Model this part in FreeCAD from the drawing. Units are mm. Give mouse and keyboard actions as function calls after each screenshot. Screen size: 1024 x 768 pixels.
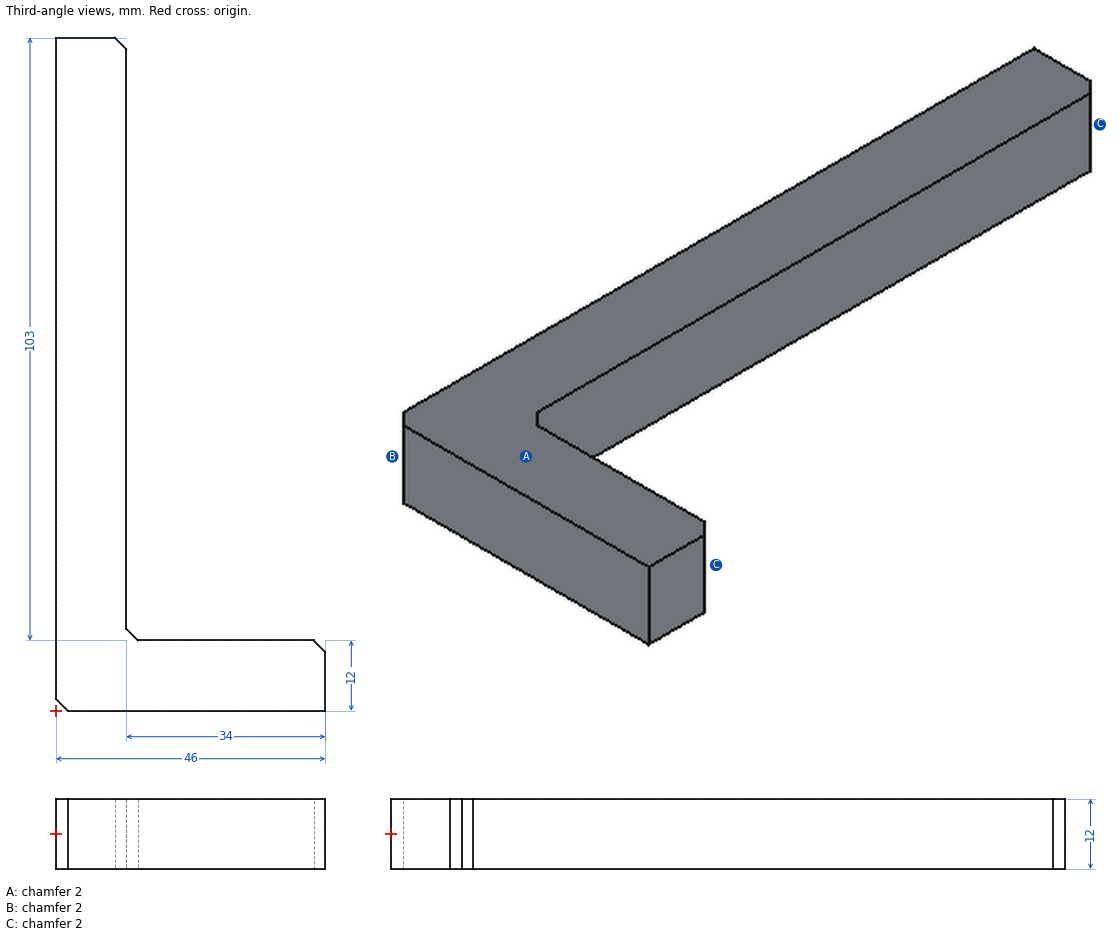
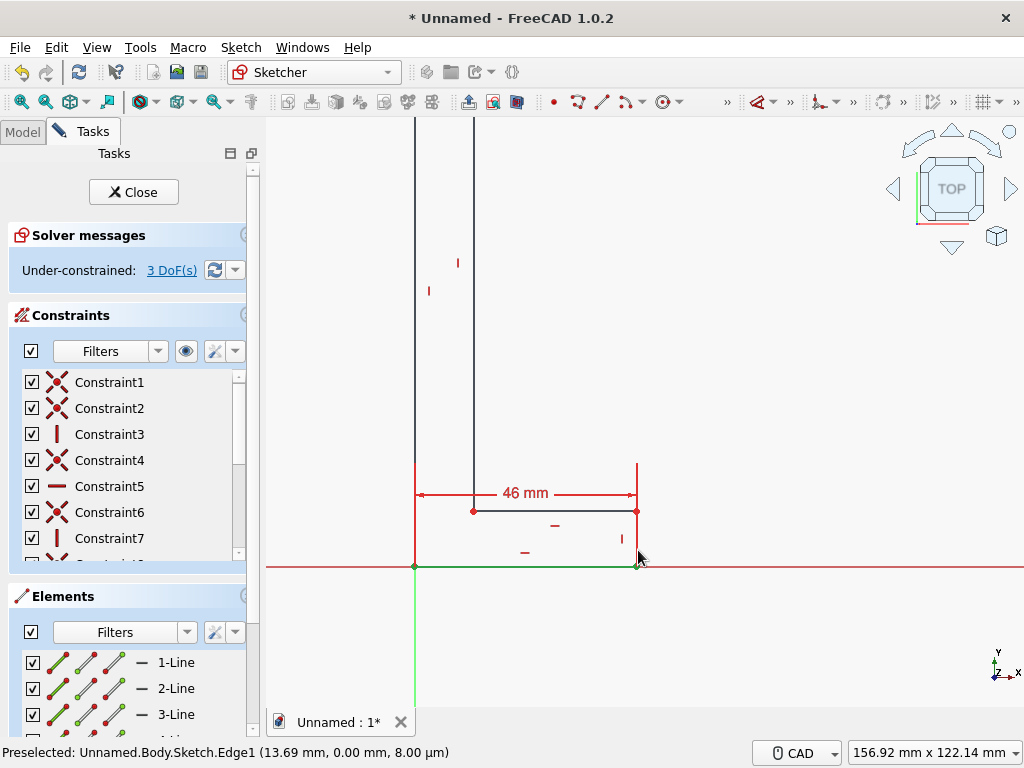
click(637, 550)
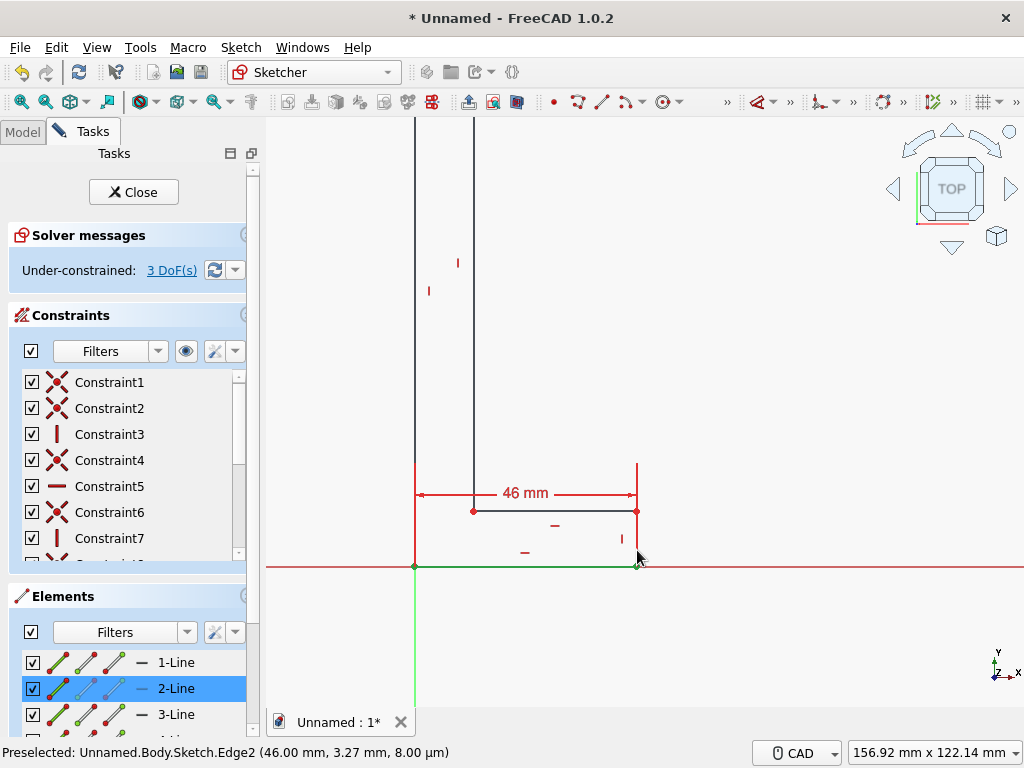
key(i)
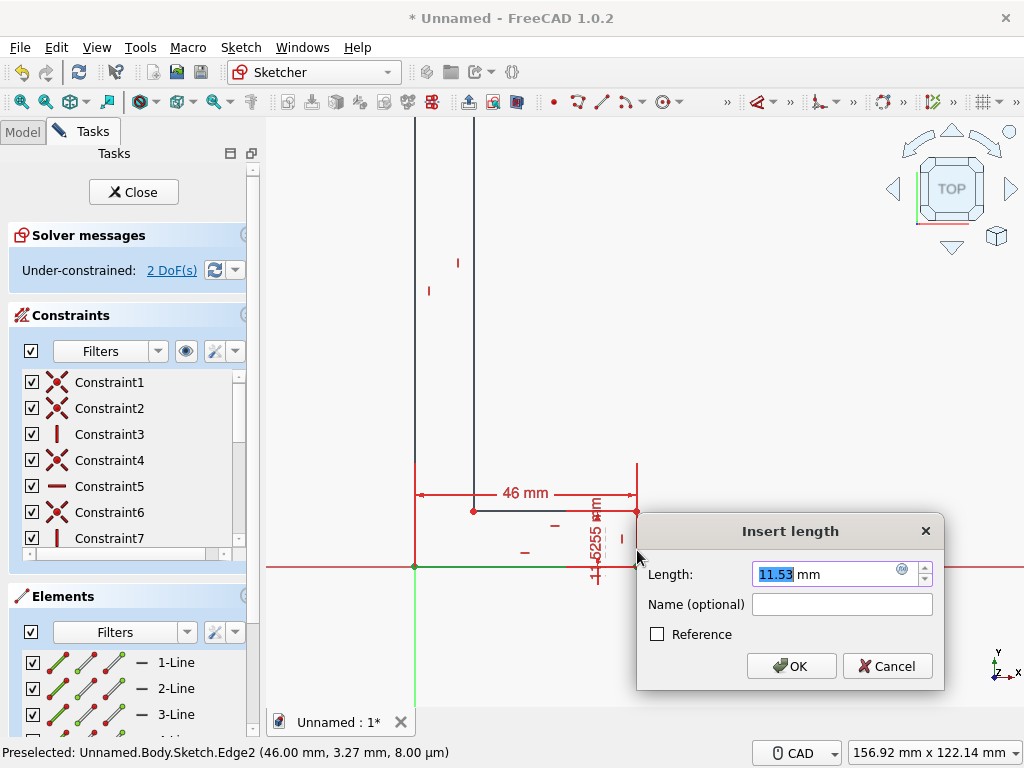
text(12)
key(Return)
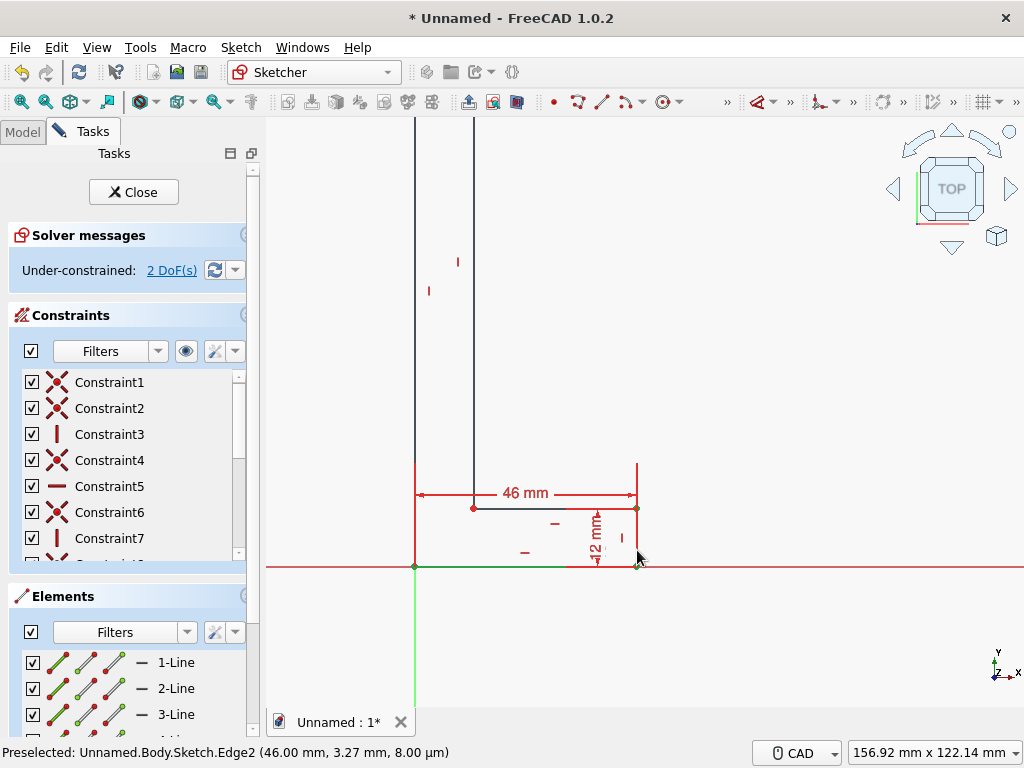
click(588, 509)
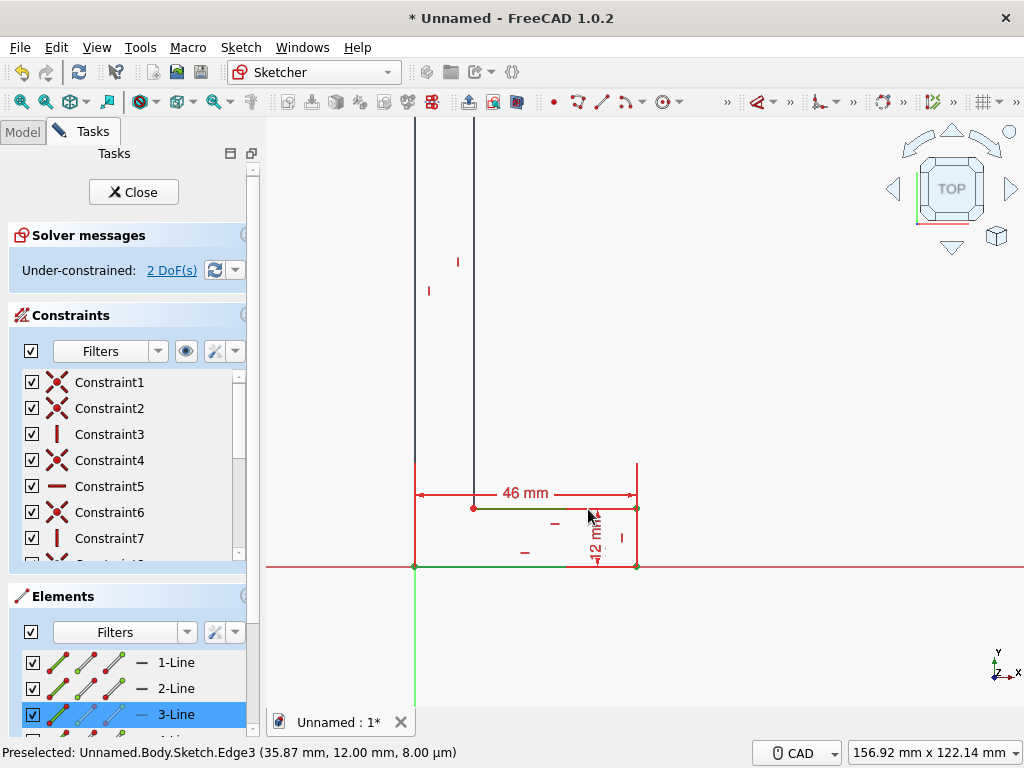
key(l)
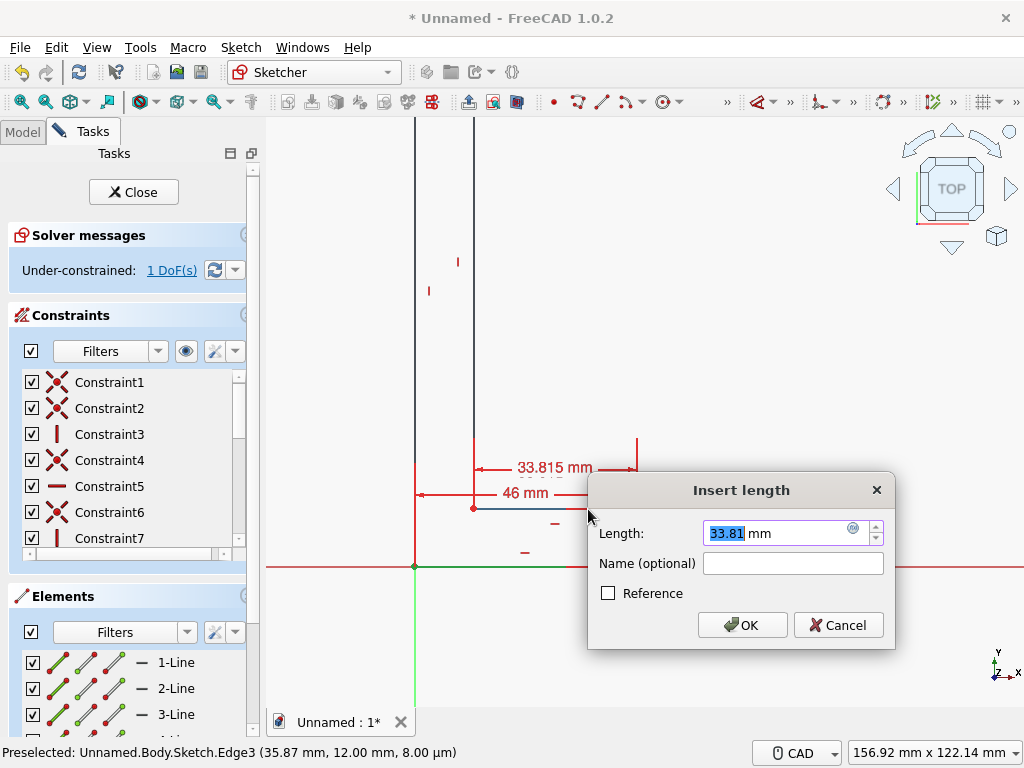
text(34)
key(Return)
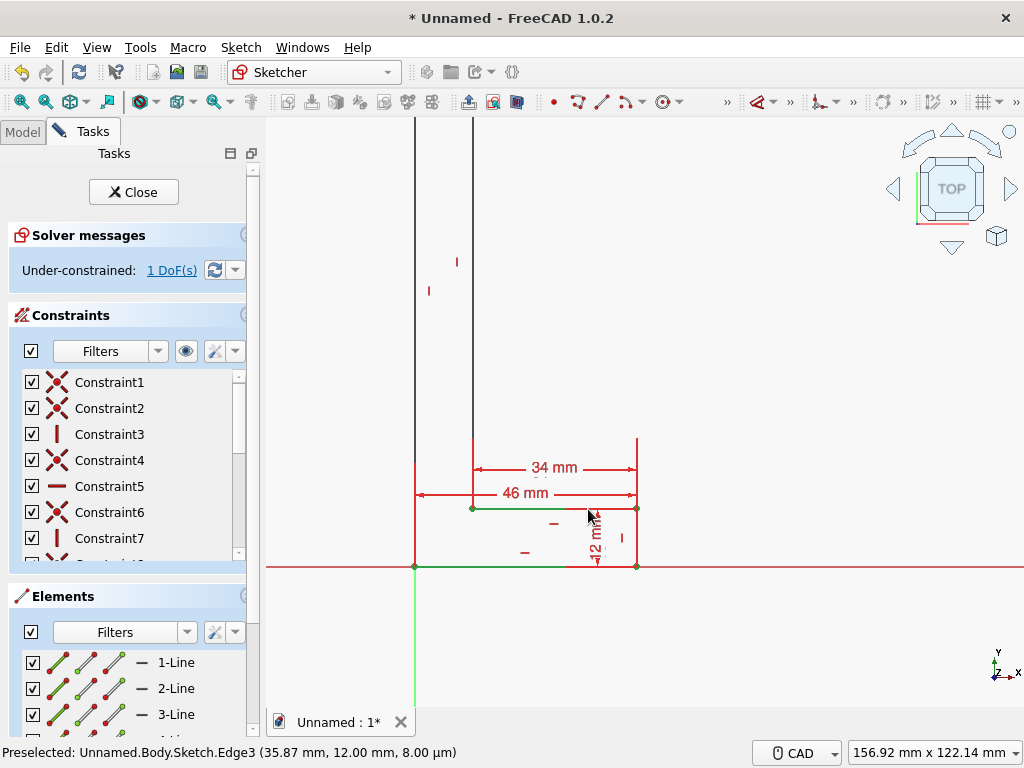
click(473, 360)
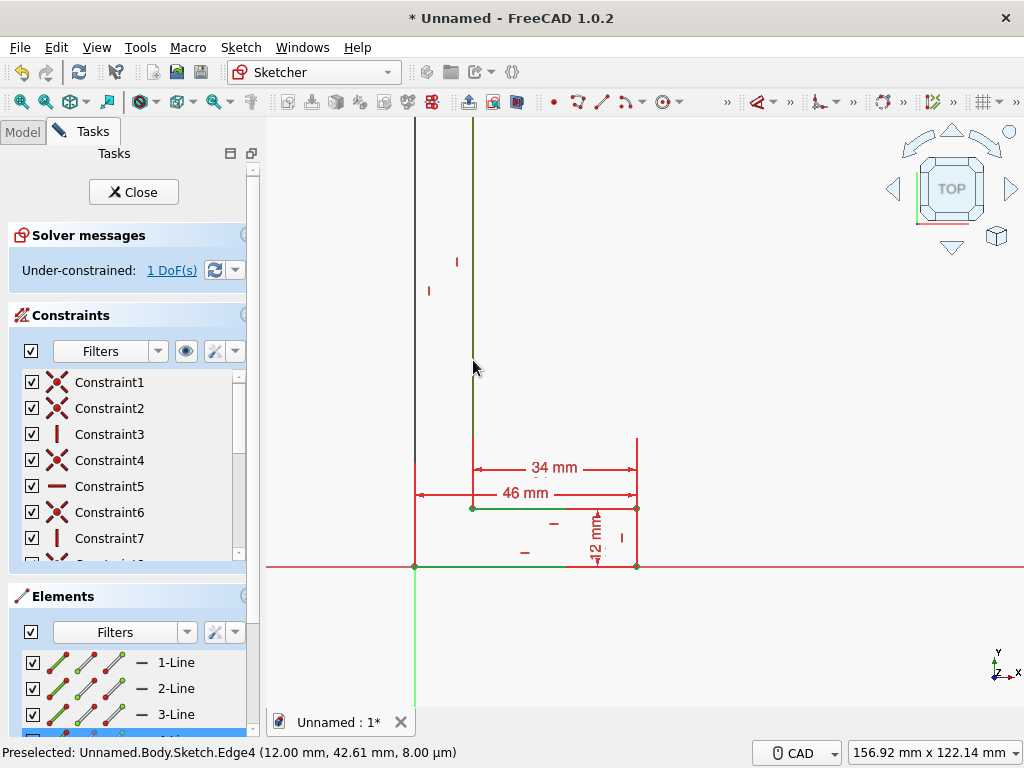
click(776, 102)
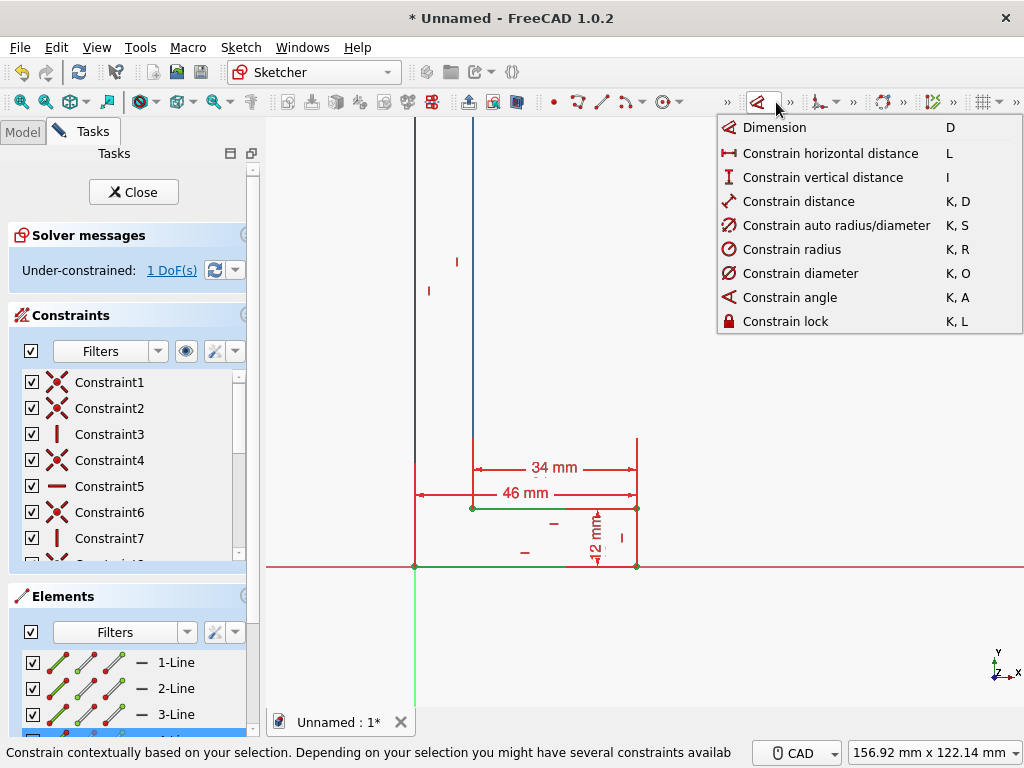
click(870, 177)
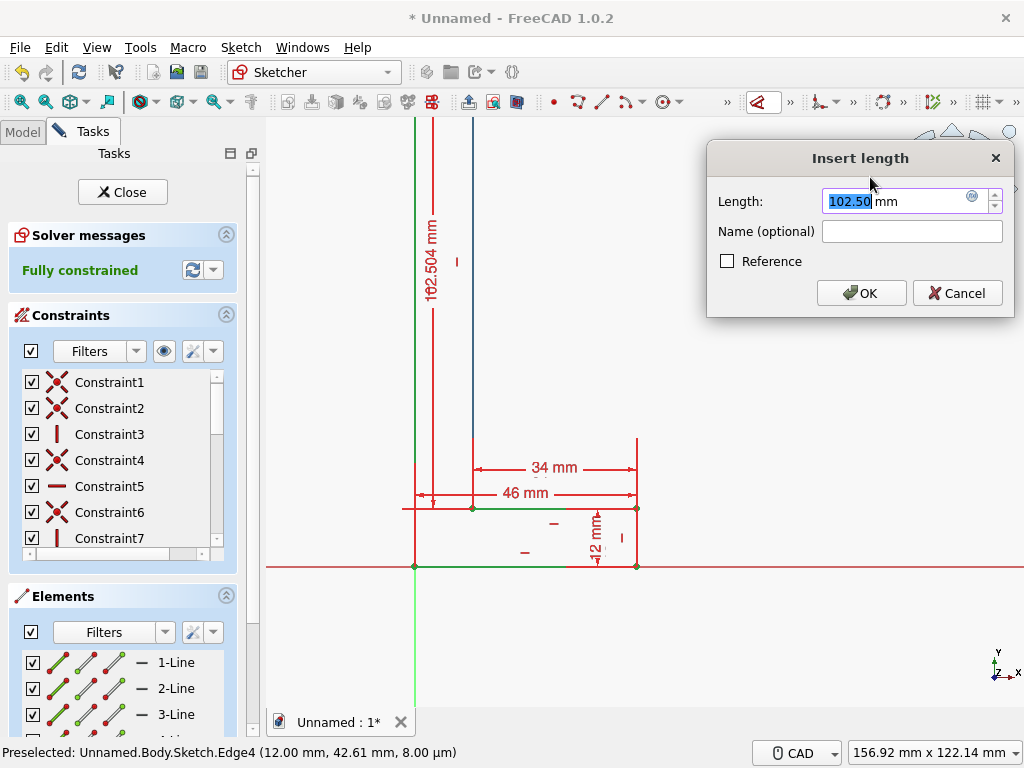
text(103)
key(Return)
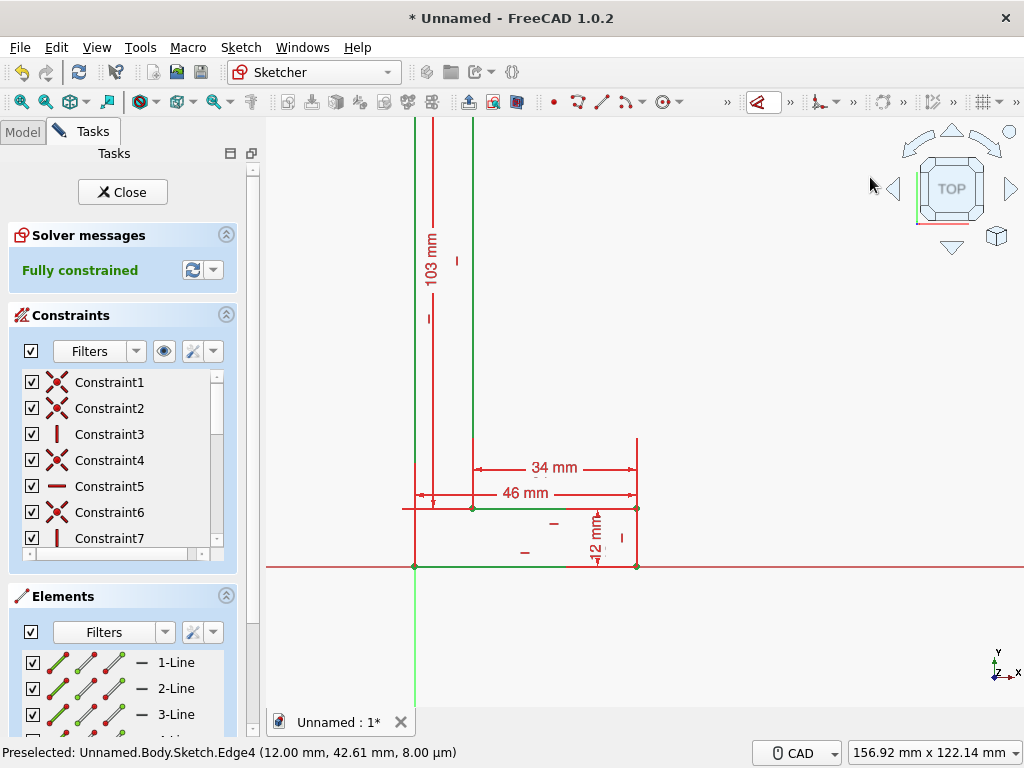
click(123, 192)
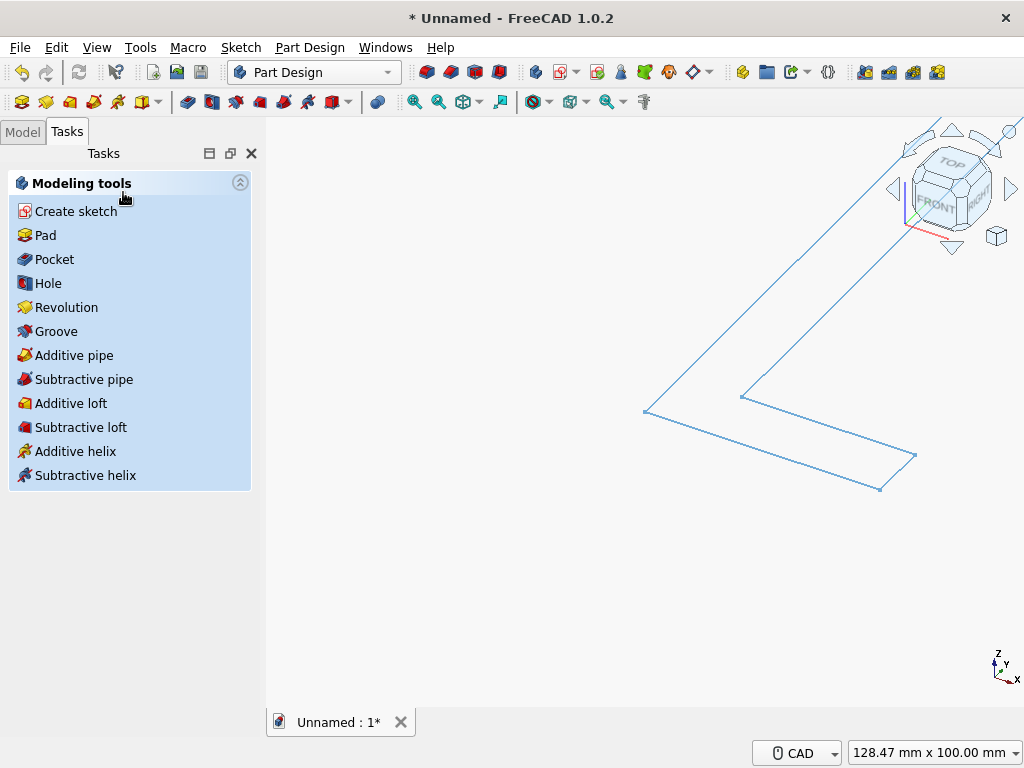
click(22, 102)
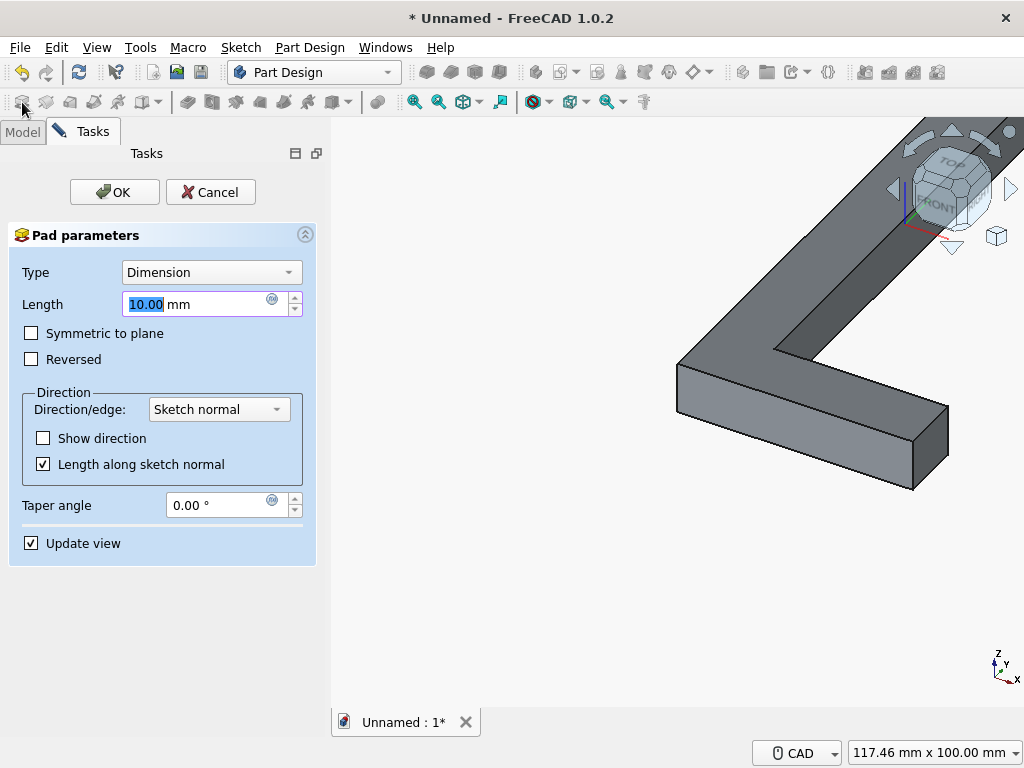
text(12)
key(Tab)